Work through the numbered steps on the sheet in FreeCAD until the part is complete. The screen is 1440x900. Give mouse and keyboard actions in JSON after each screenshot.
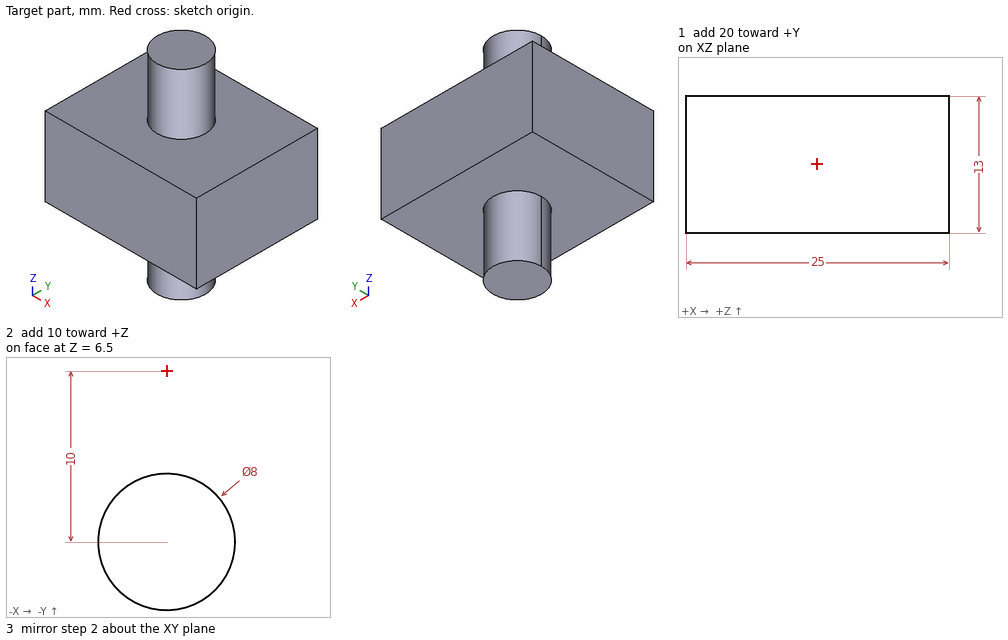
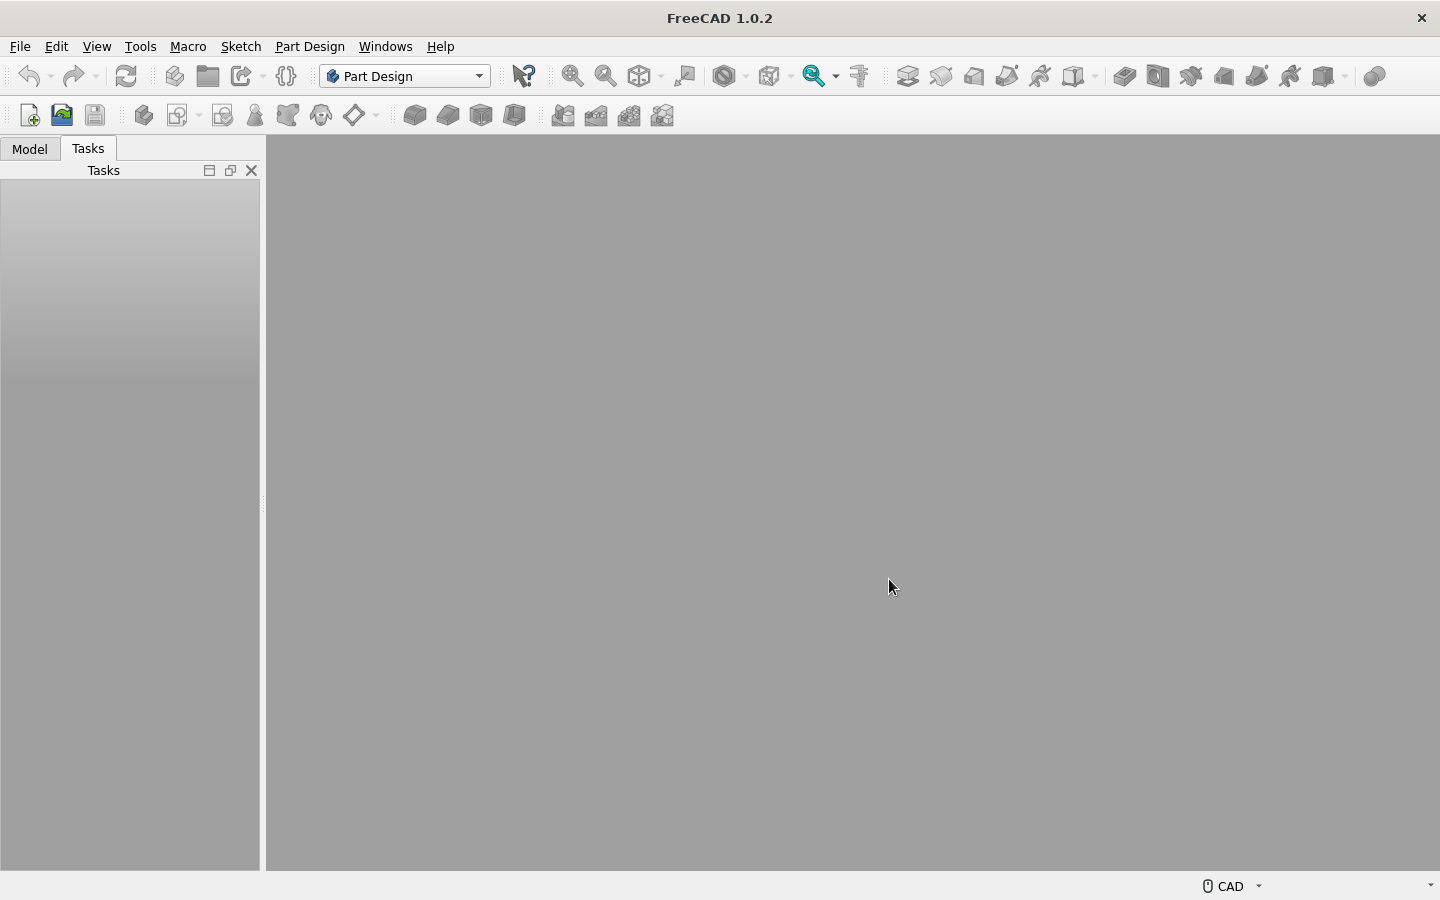
{"action": "key", "text": "ctrl+n"}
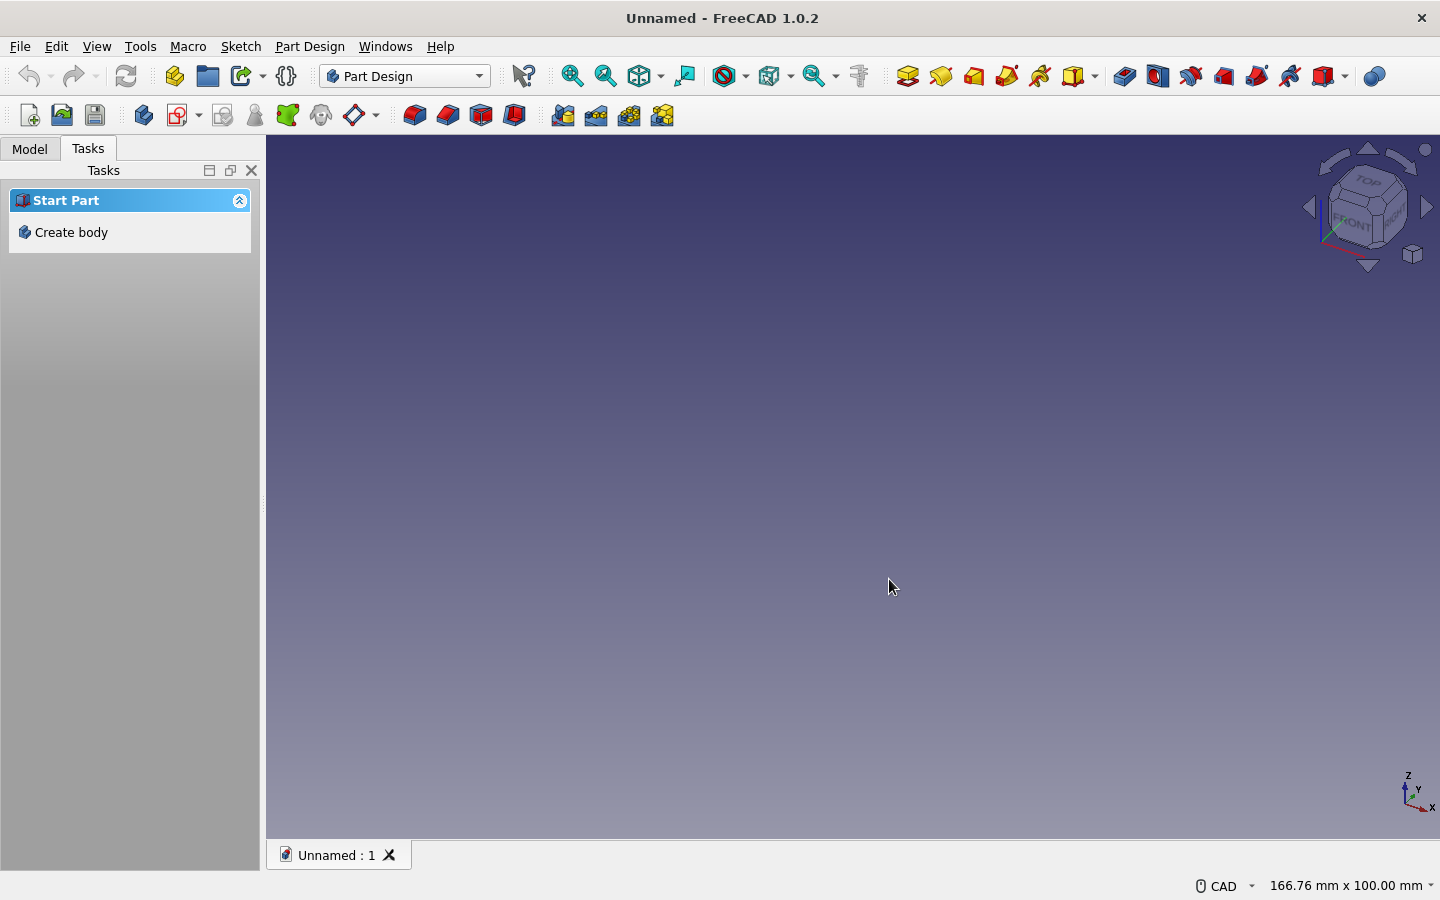
{"action": "left_click", "coordinate": [176, 116]}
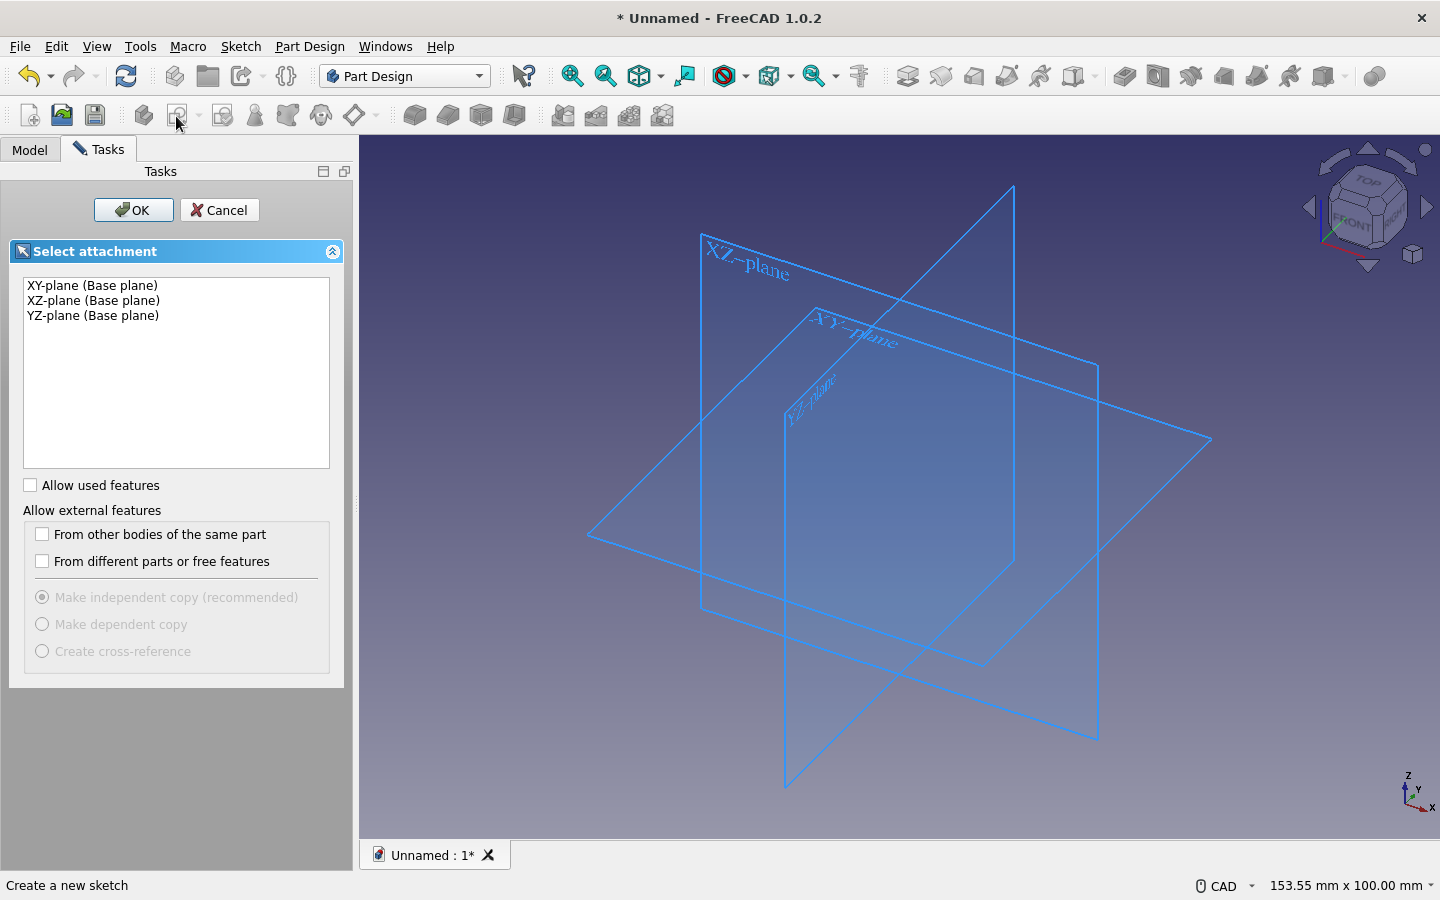
{"action": "left_click", "coordinate": [84, 300]}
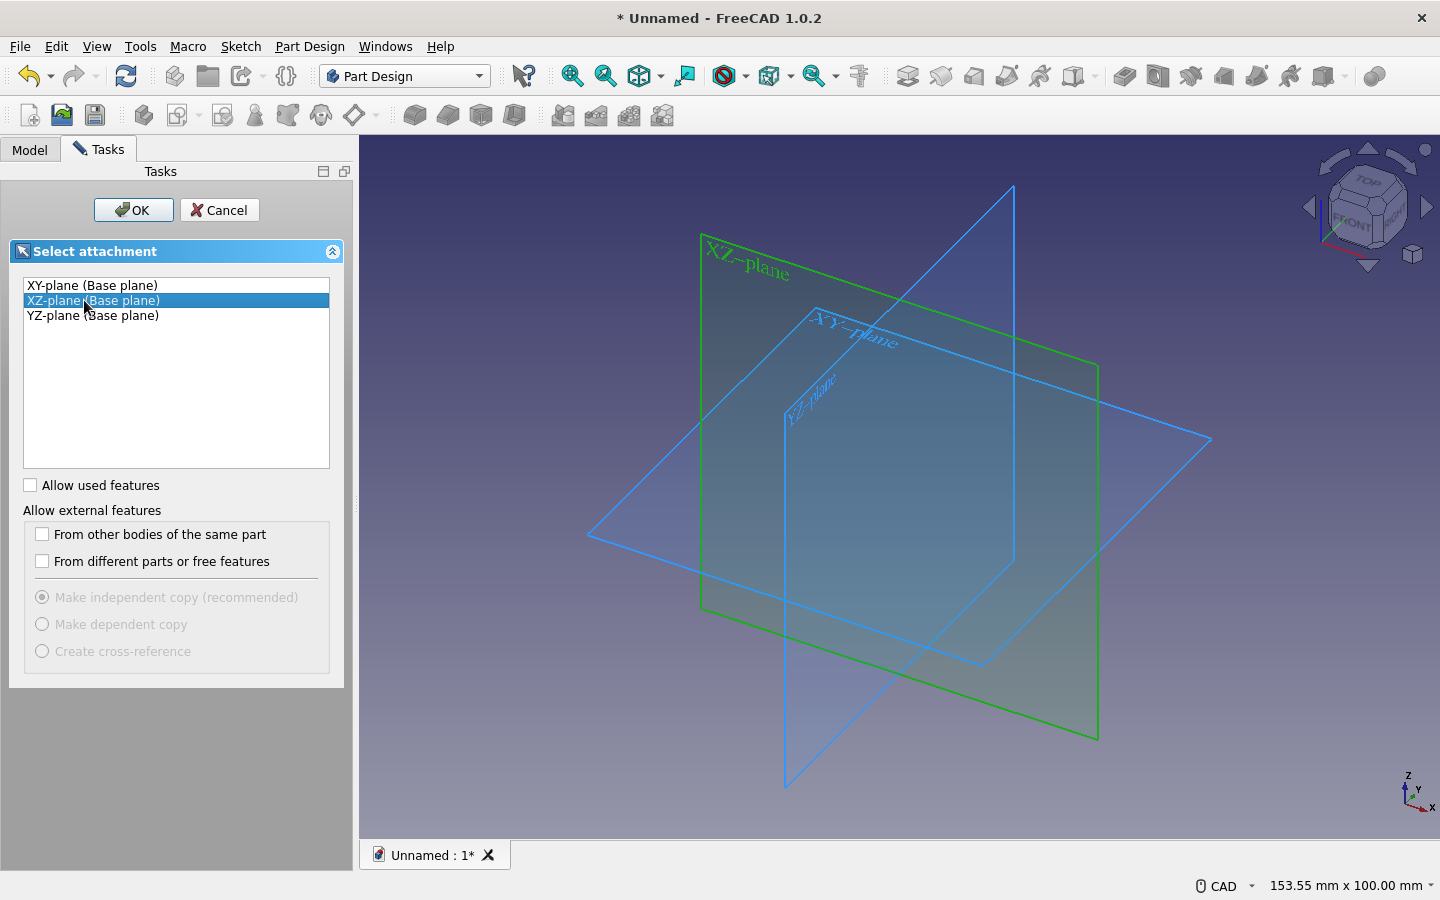
{"action": "left_click", "coordinate": [134, 210]}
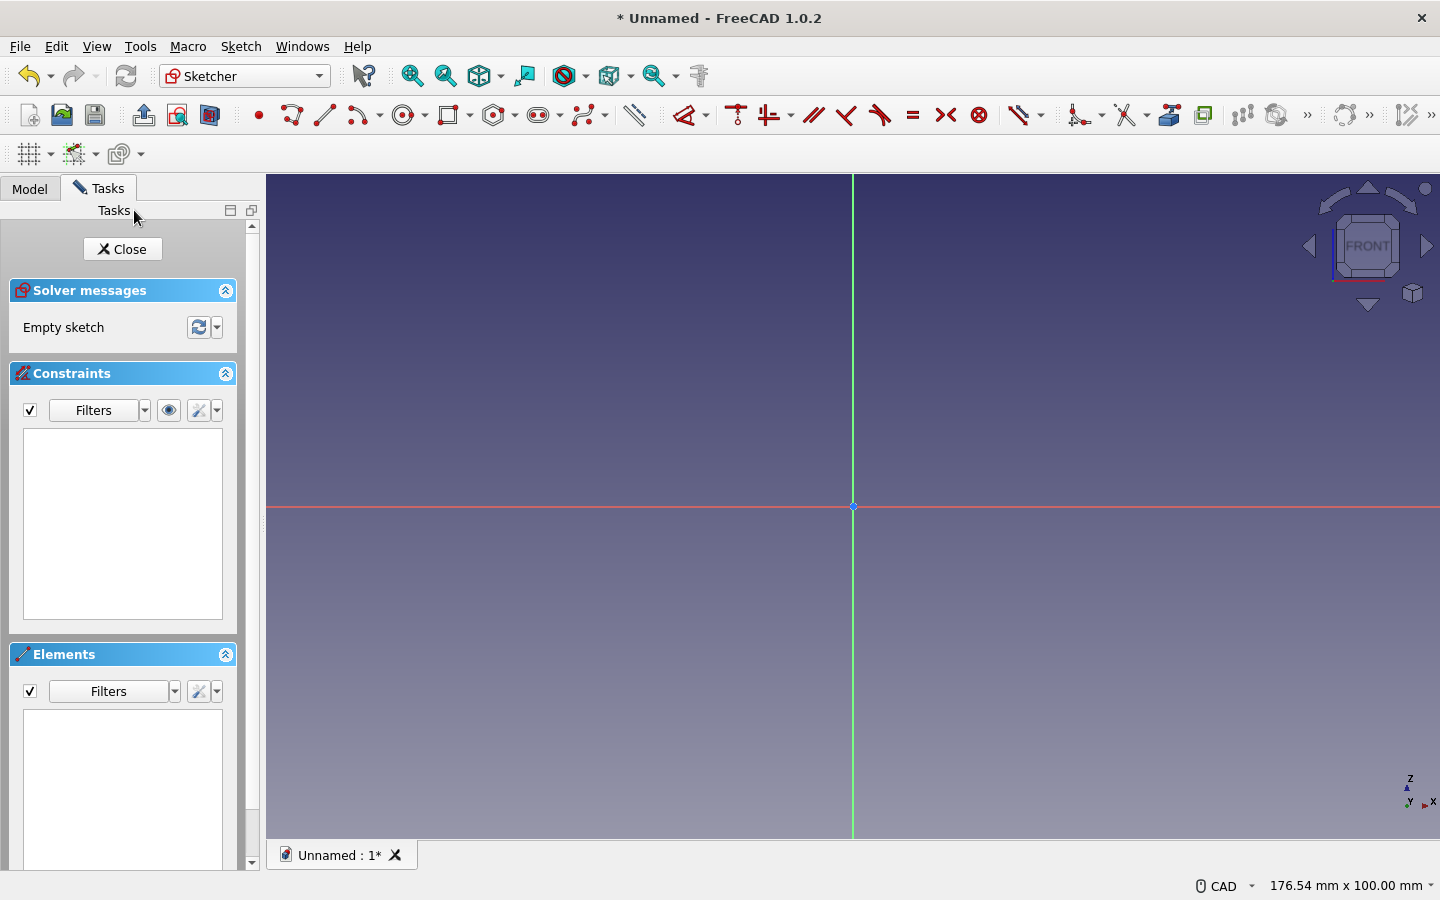
{"action": "scroll", "coordinate": [875, 507], "scroll_direction": "up", "scroll_amount": 7}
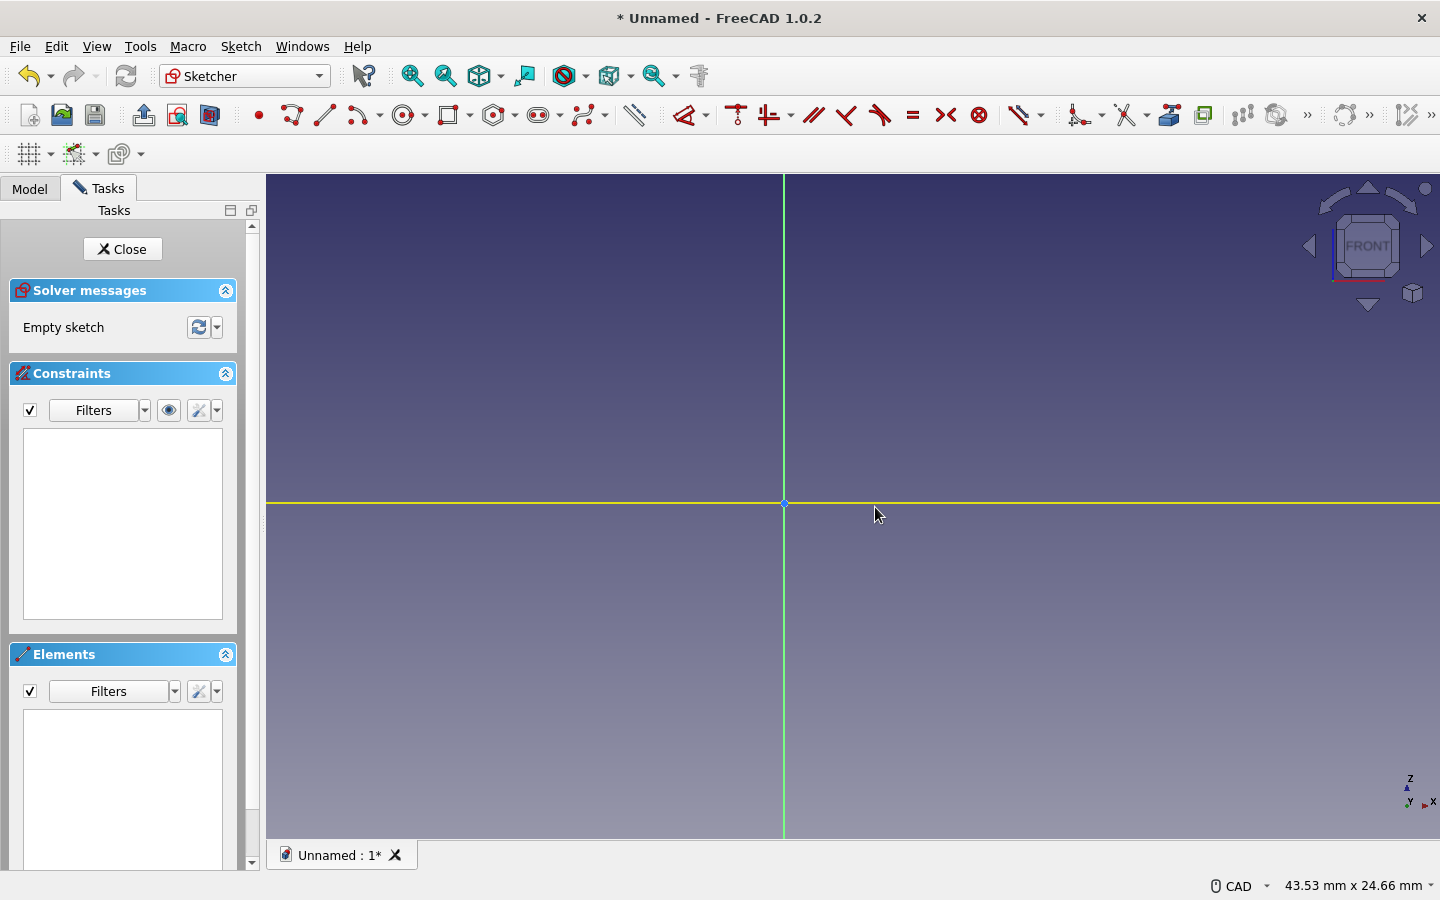
{"action": "key", "text": "g v"}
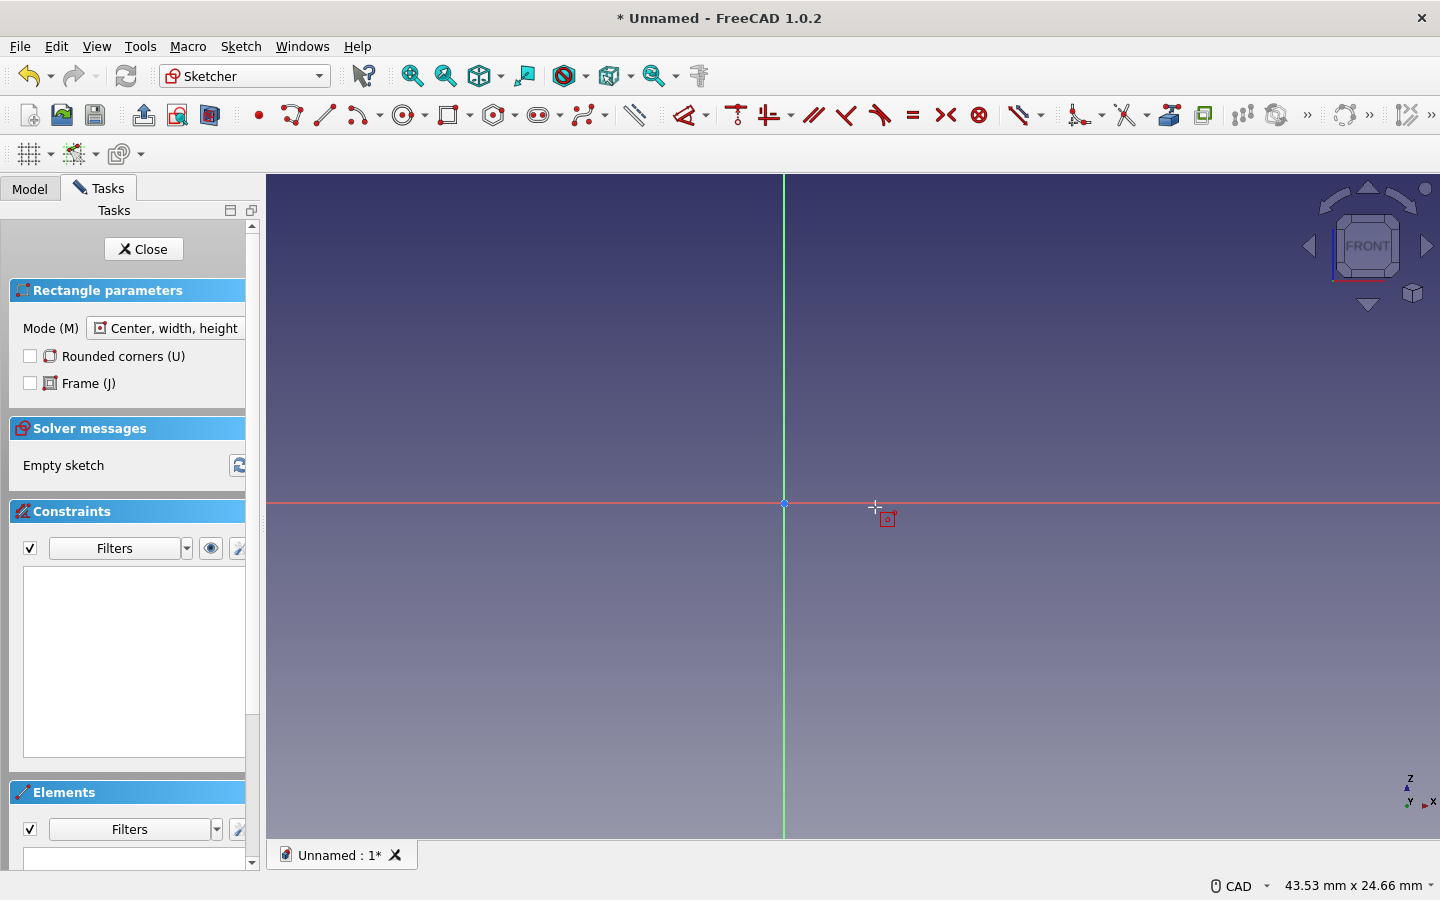
{"action": "left_click", "coordinate": [784, 503]}
{"action": "left_click", "coordinate": [1121, 328]}
{"action": "key", "text": "Escape"}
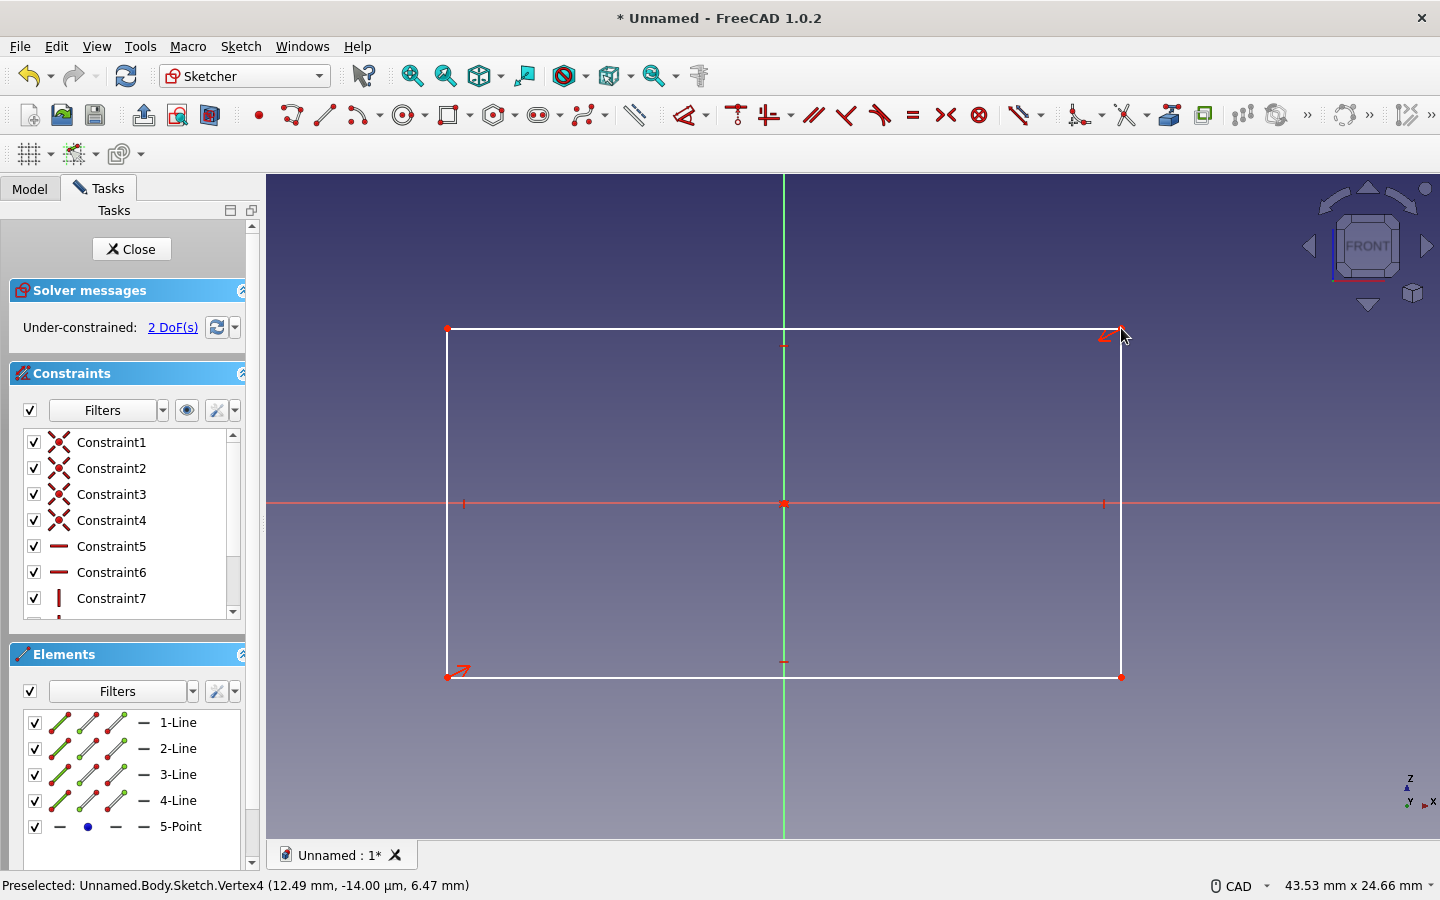
{"action": "left_click", "coordinate": [649, 678]}